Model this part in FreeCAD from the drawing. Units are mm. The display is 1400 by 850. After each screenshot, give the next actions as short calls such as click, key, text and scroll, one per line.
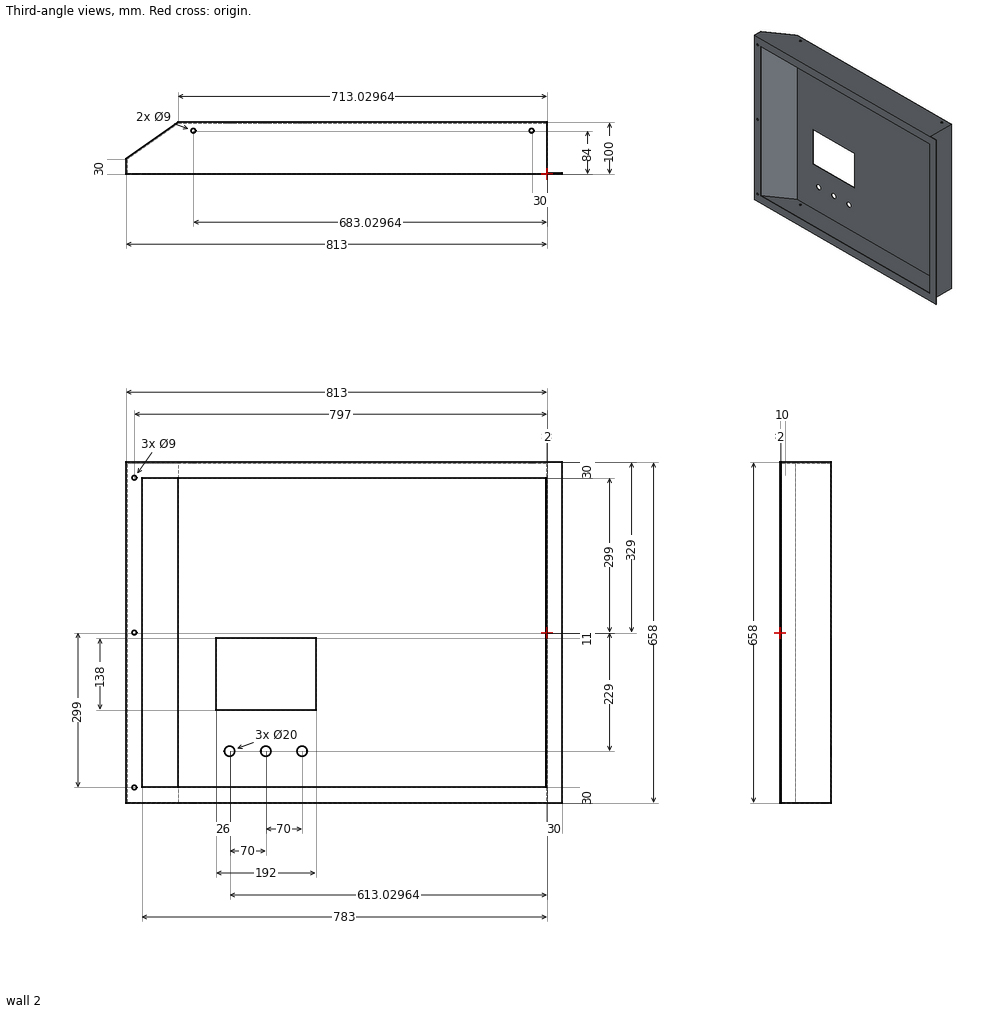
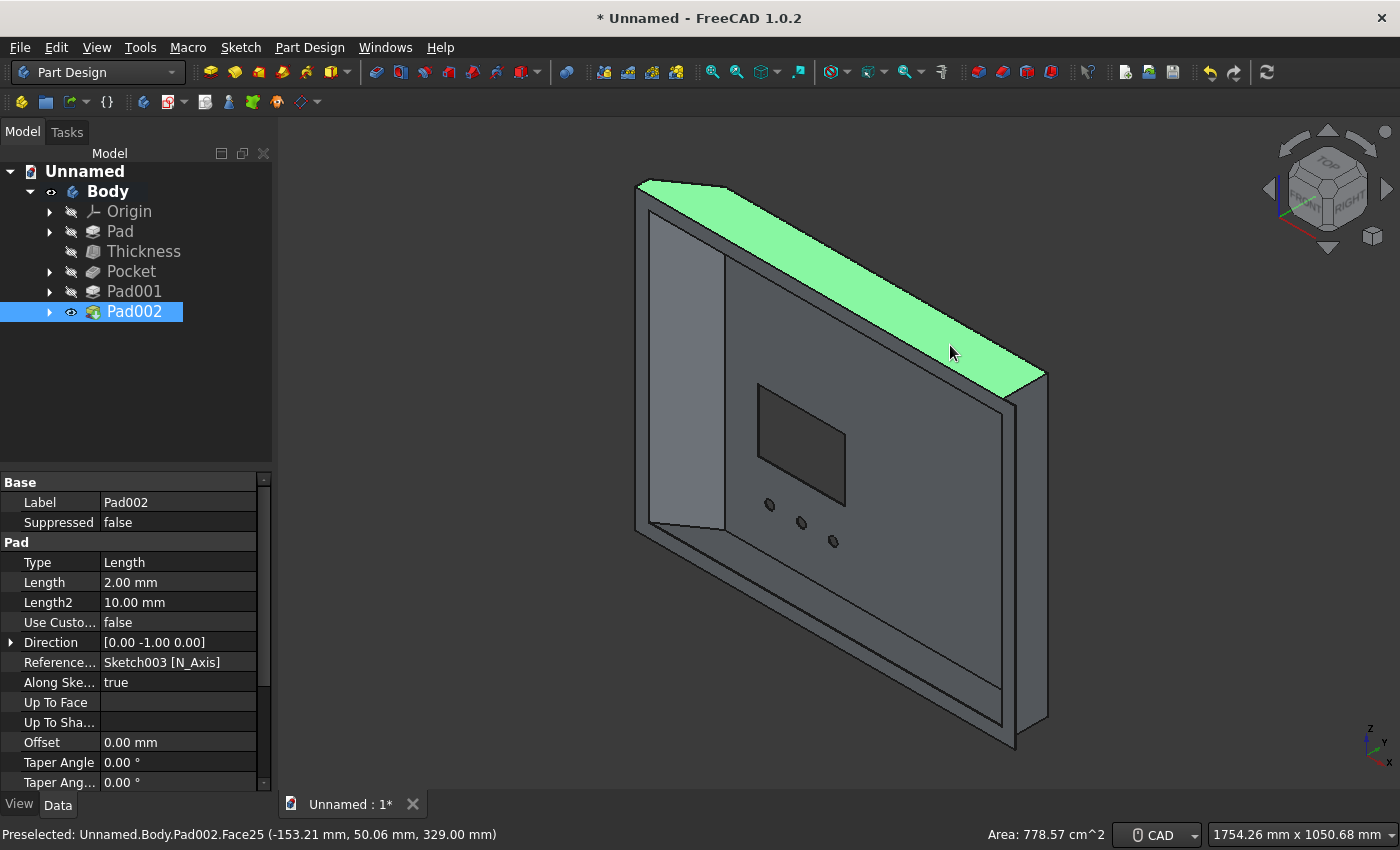
click(168, 102)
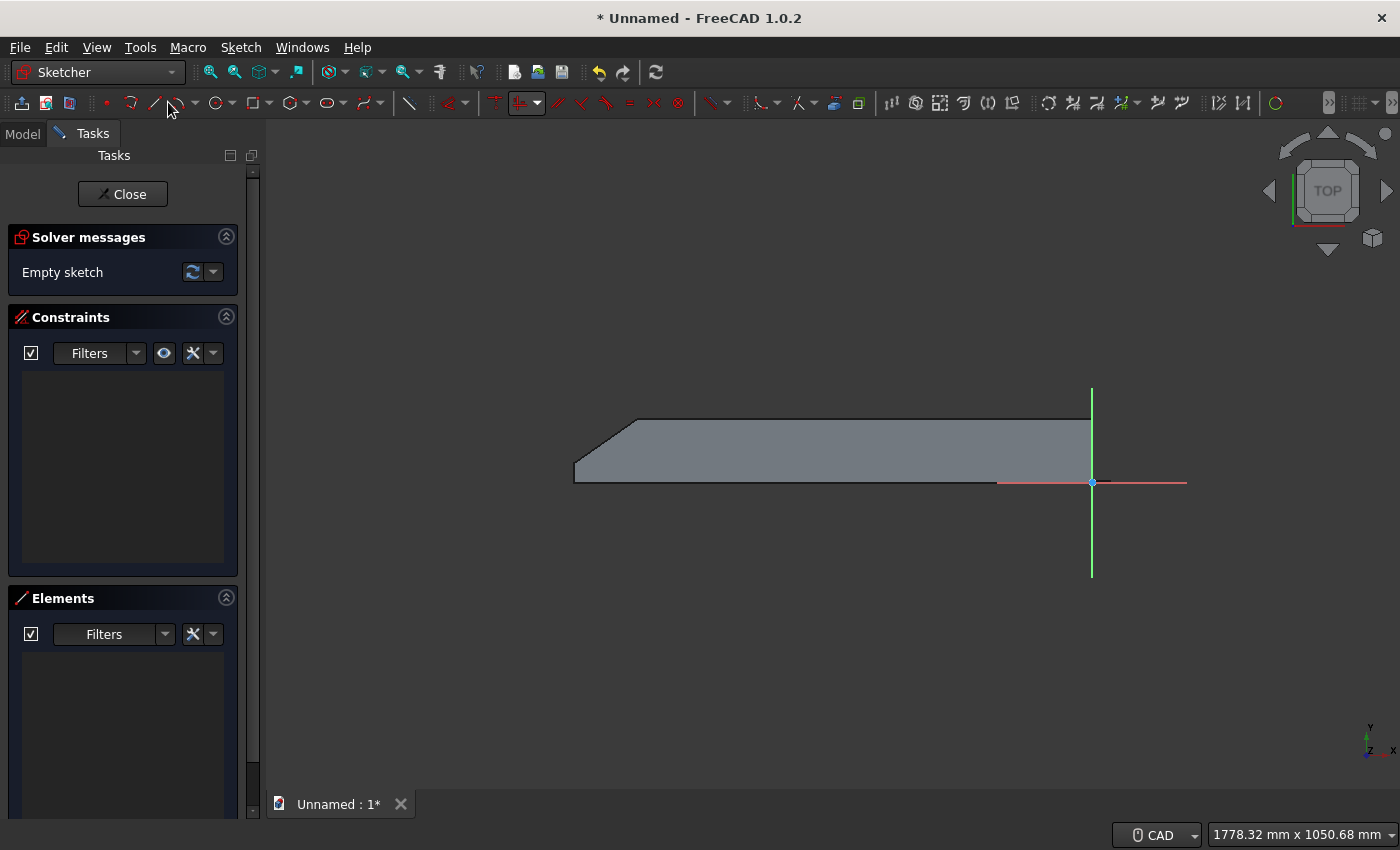
scroll(1094, 455, up, 2)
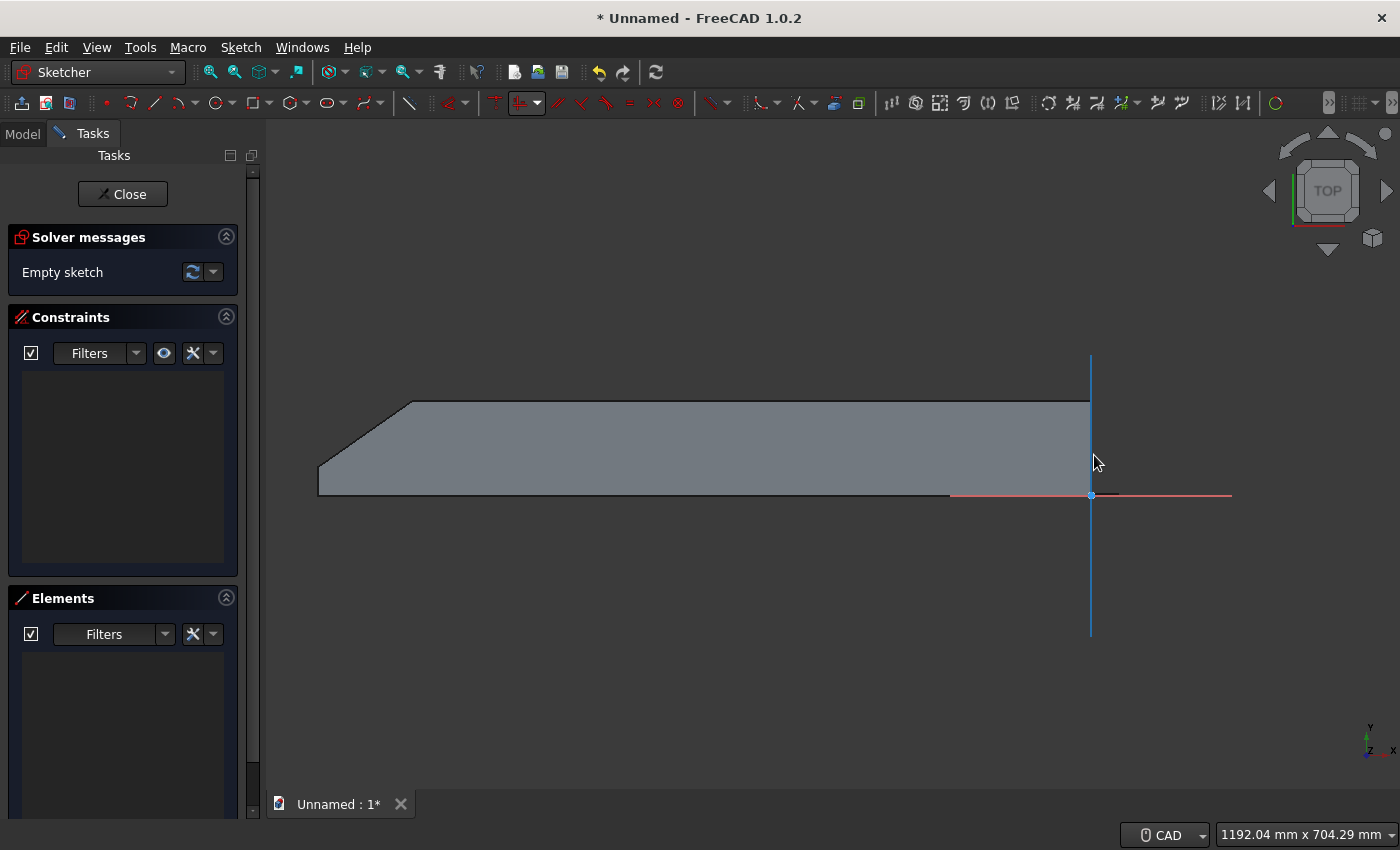
click(216, 104)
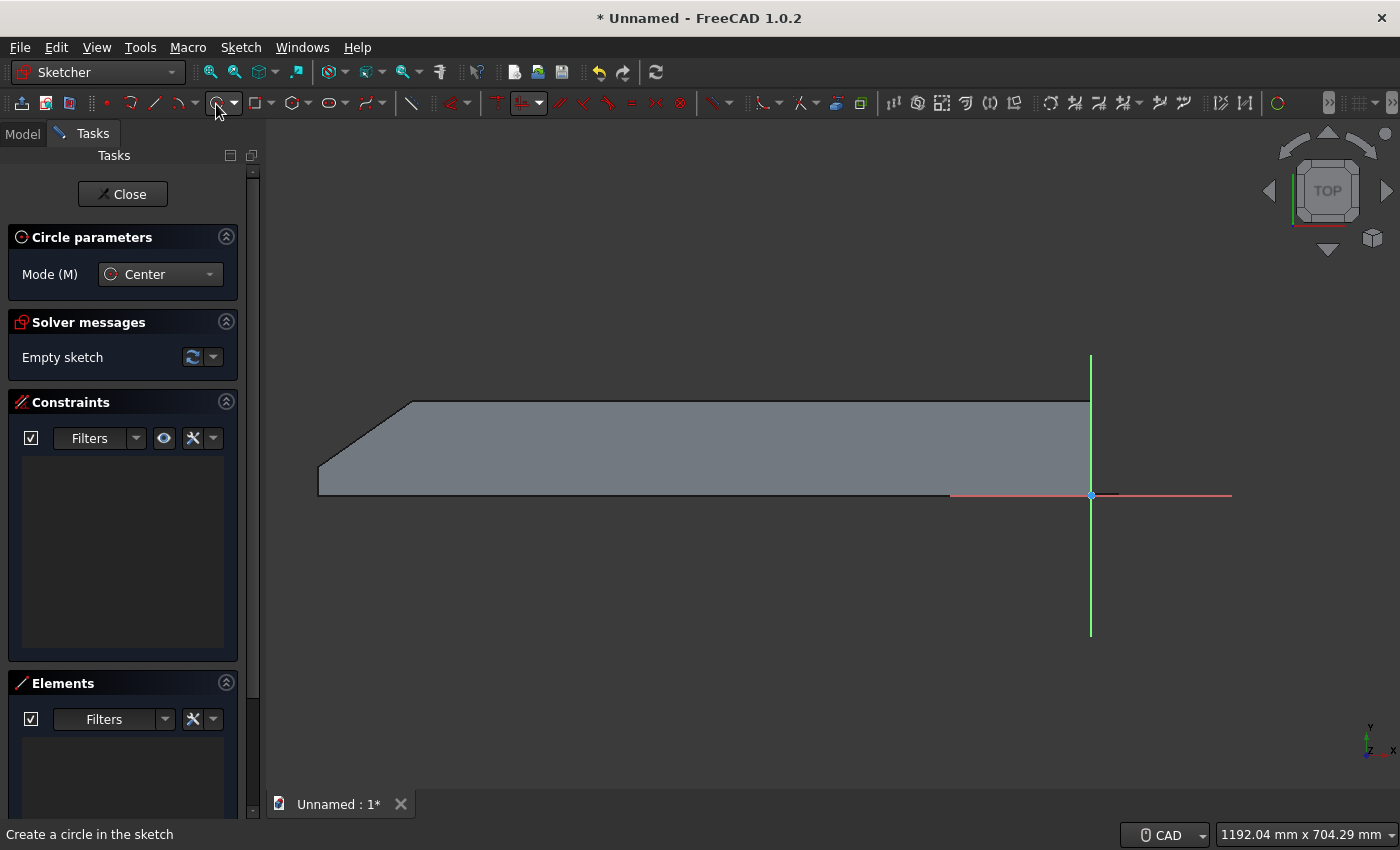
scroll(441, 416, up, 9)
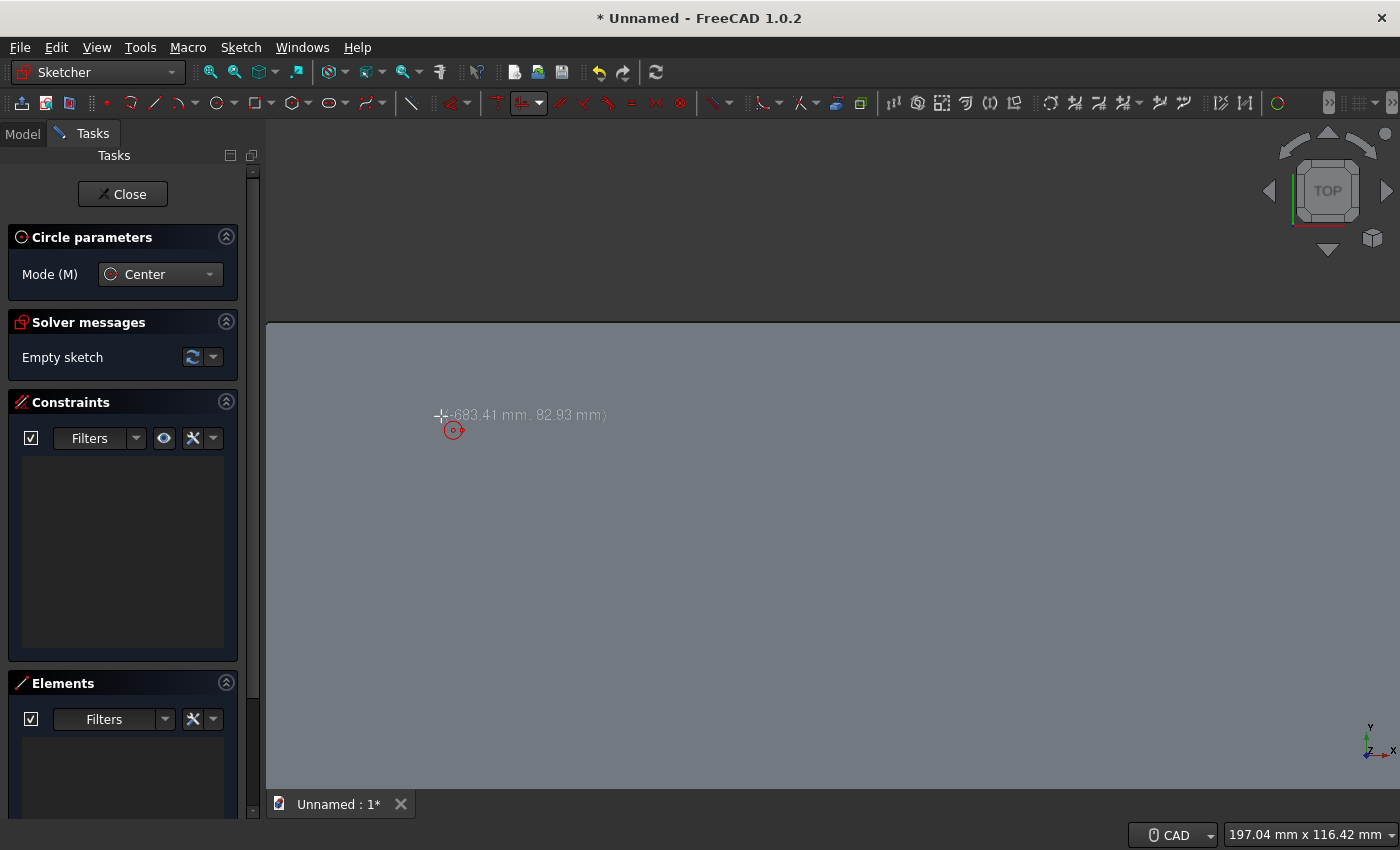
scroll(442, 417, down, 9)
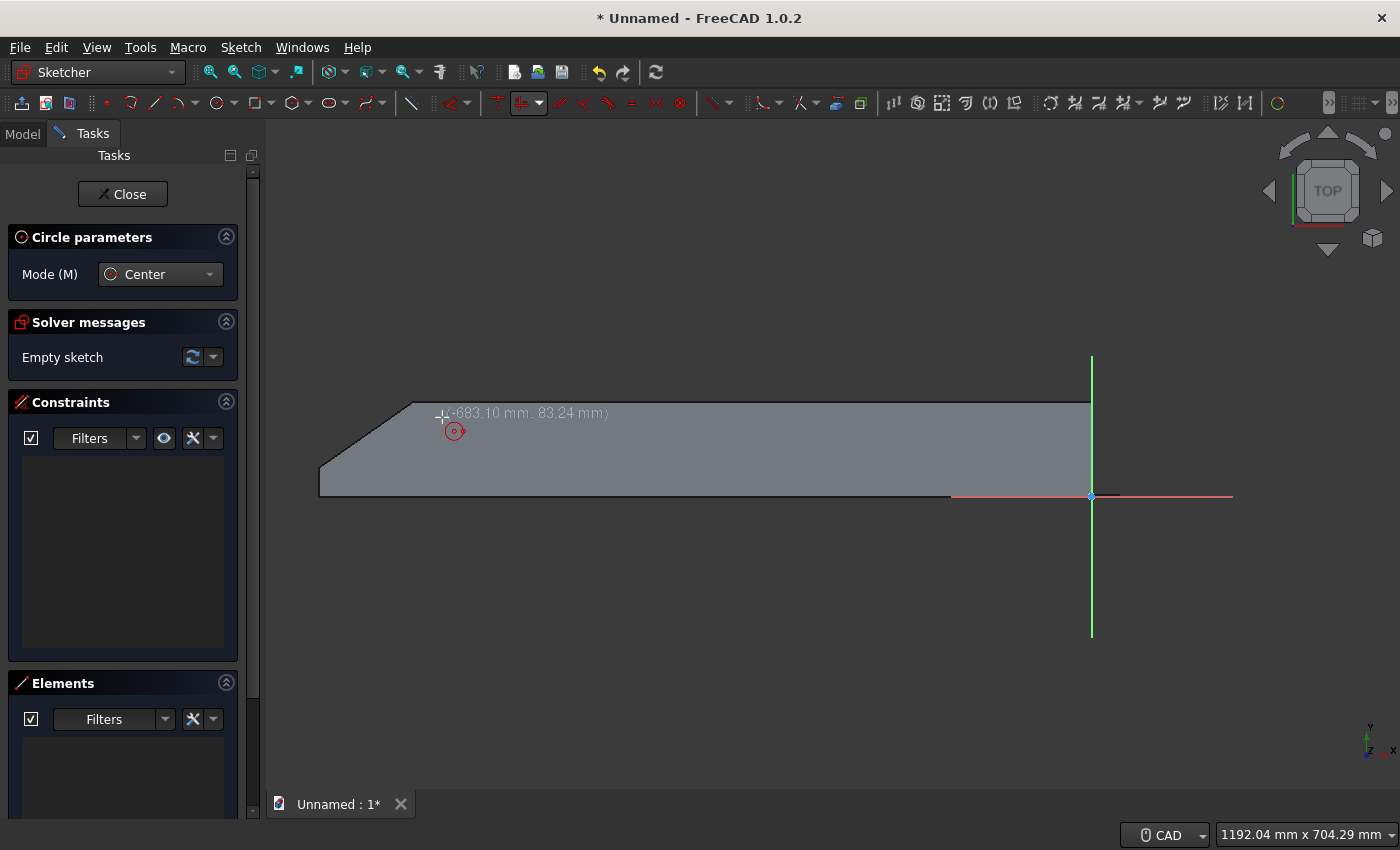
click(442, 417)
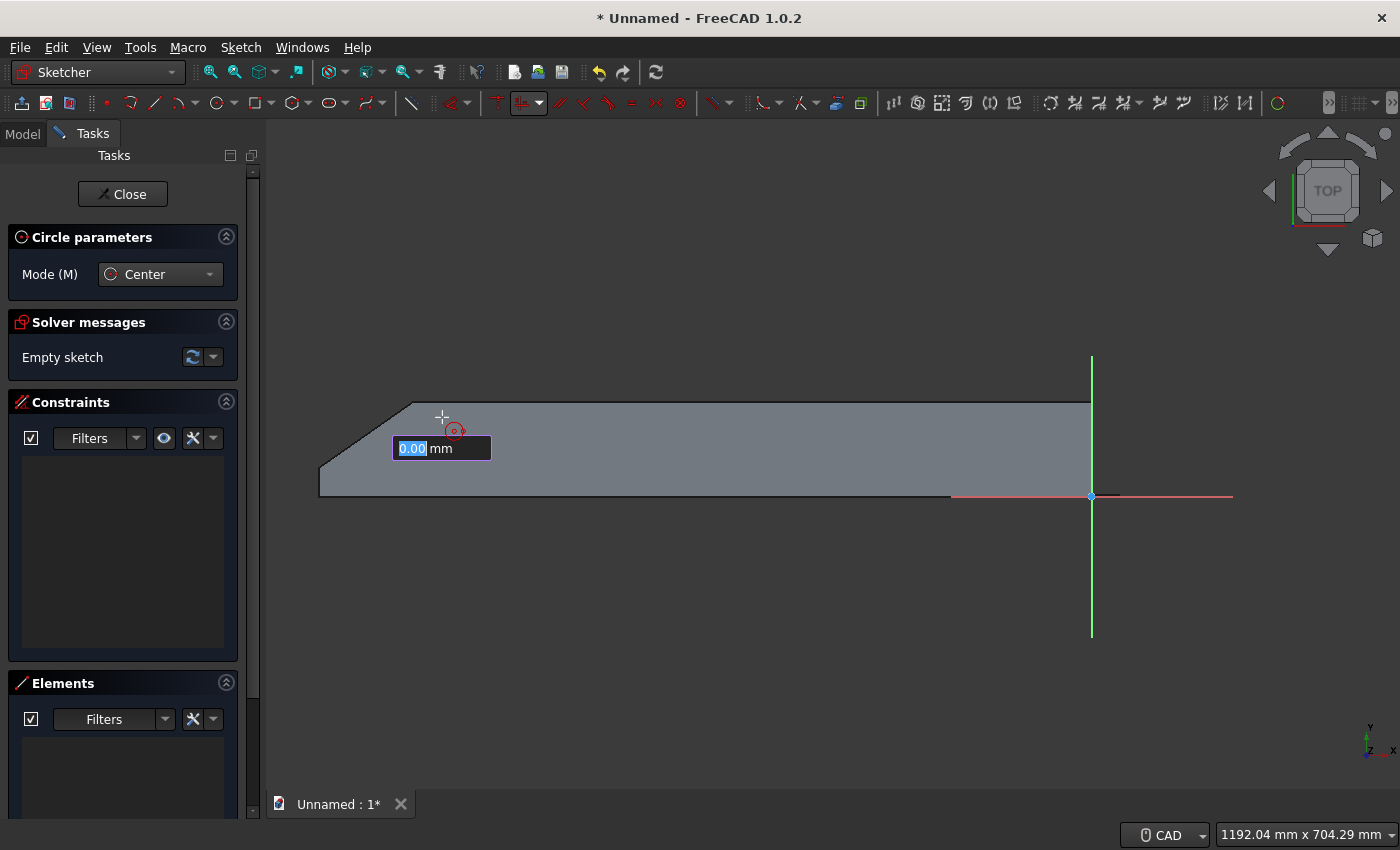
scroll(445, 414, up, 7)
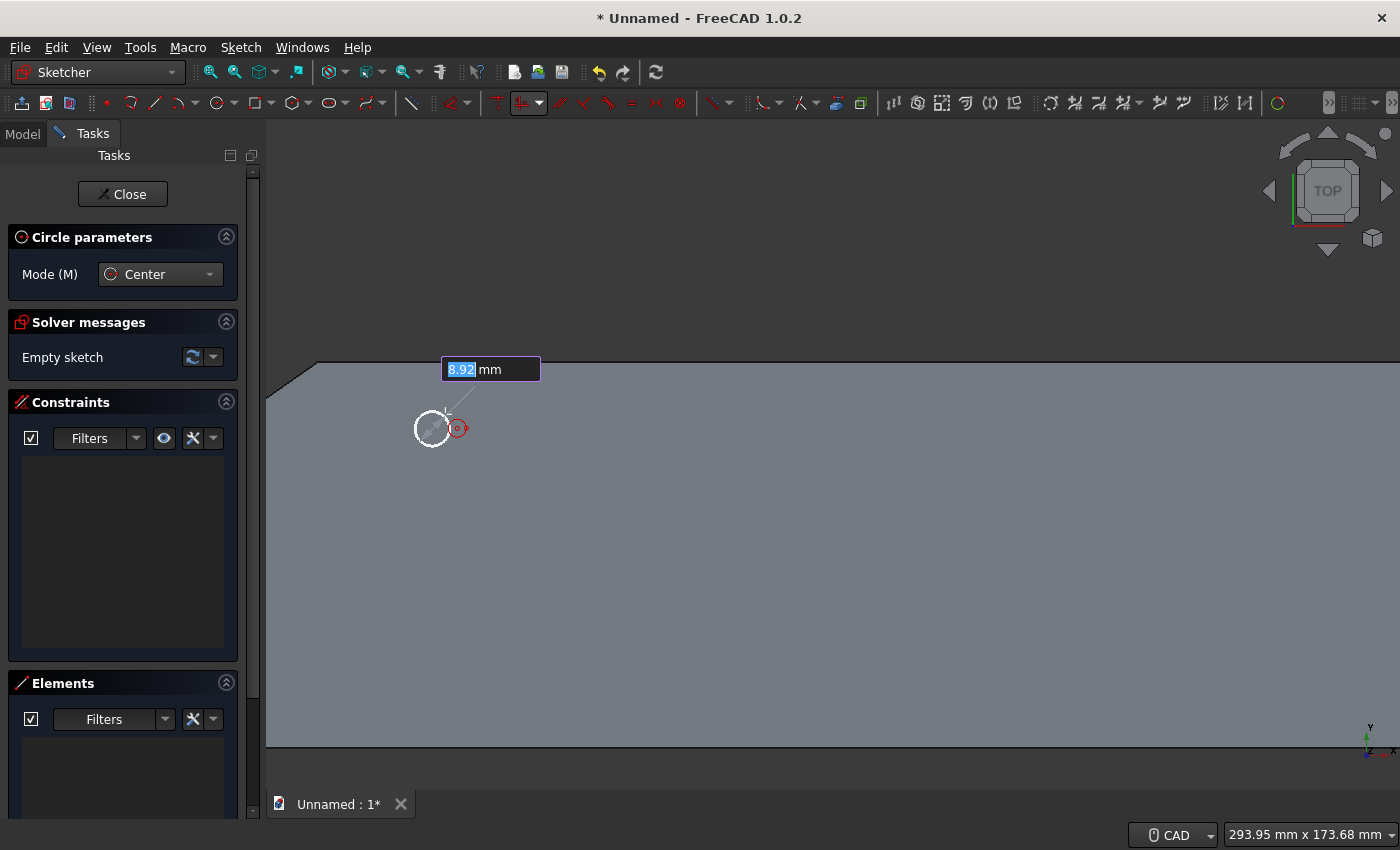
click(445, 412)